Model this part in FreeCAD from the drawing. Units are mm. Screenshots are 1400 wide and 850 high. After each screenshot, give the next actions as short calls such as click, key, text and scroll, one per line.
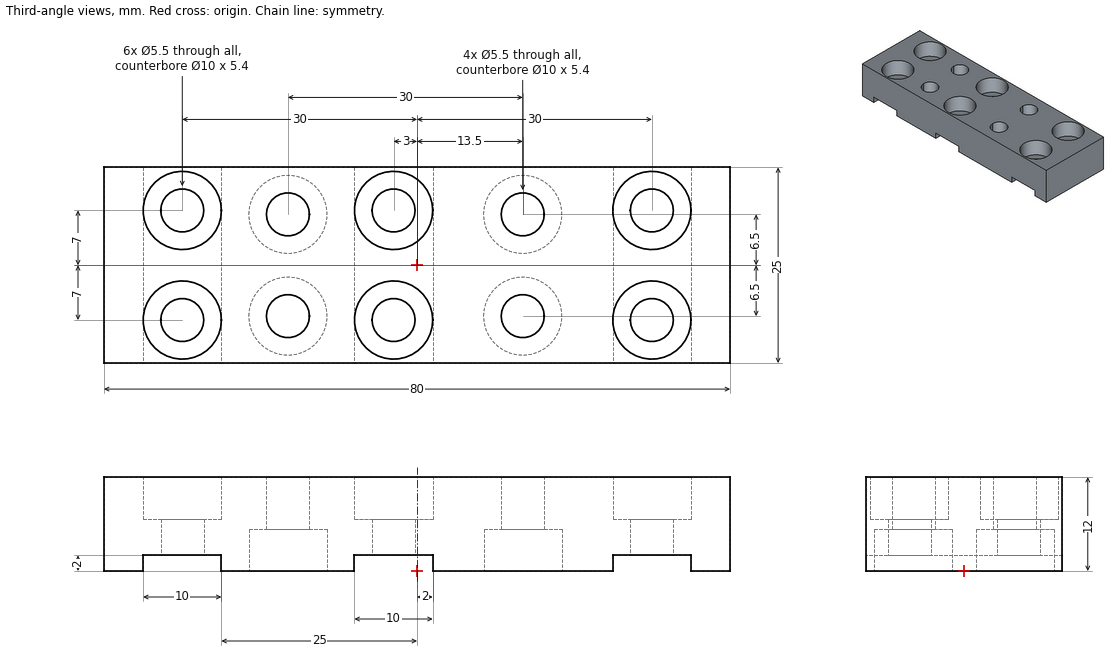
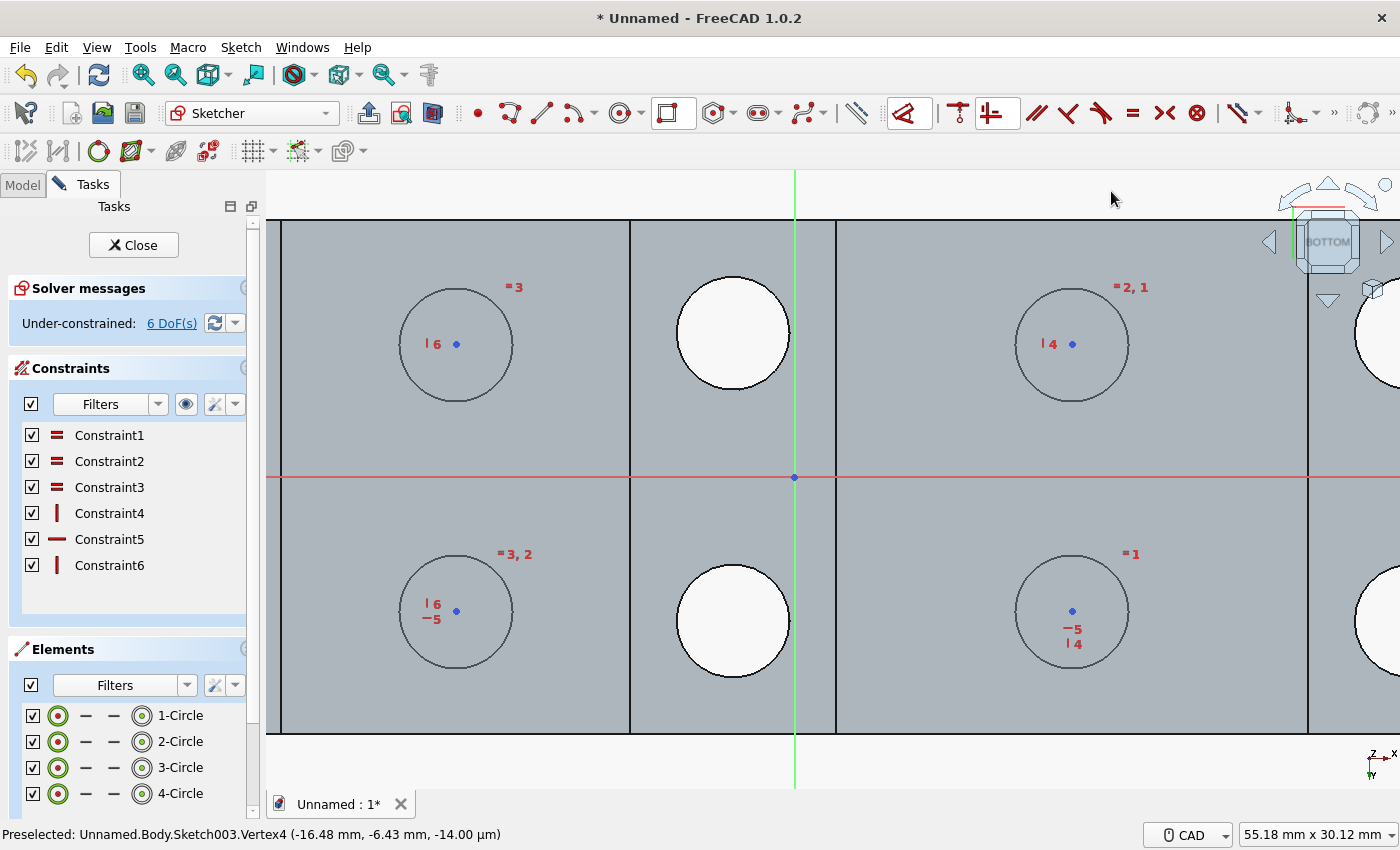
click(1072, 345)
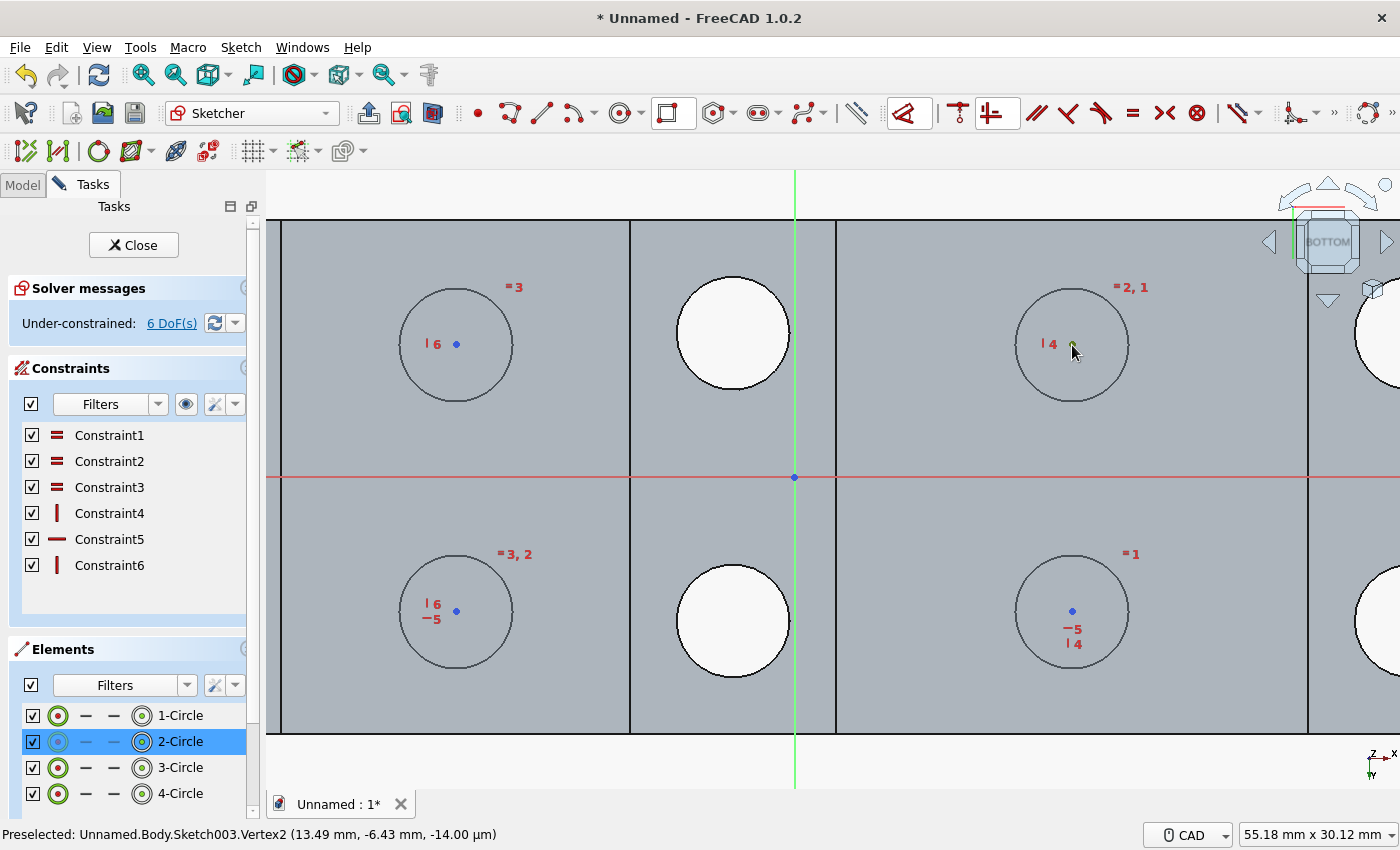
click(456, 345)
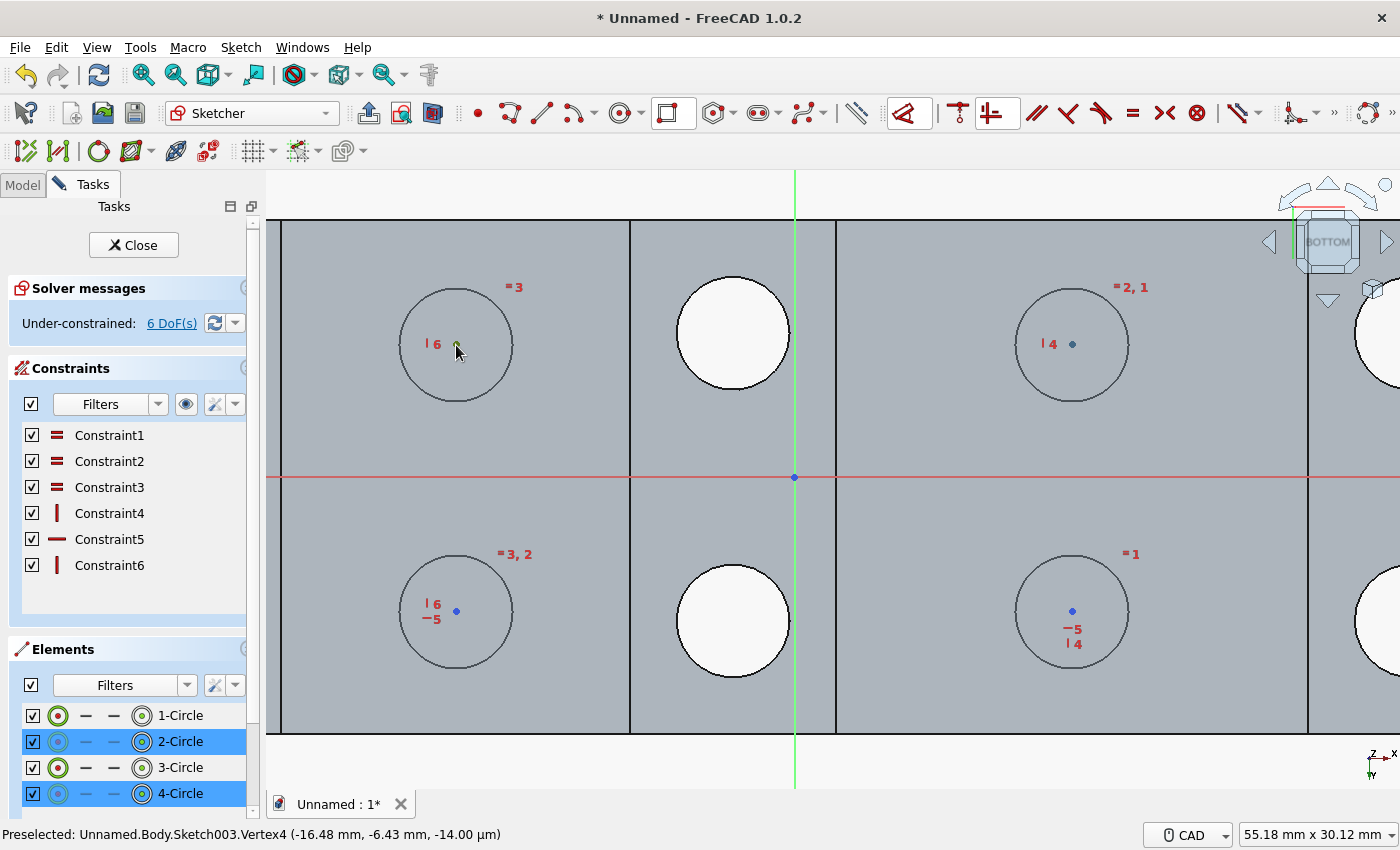
click(1014, 114)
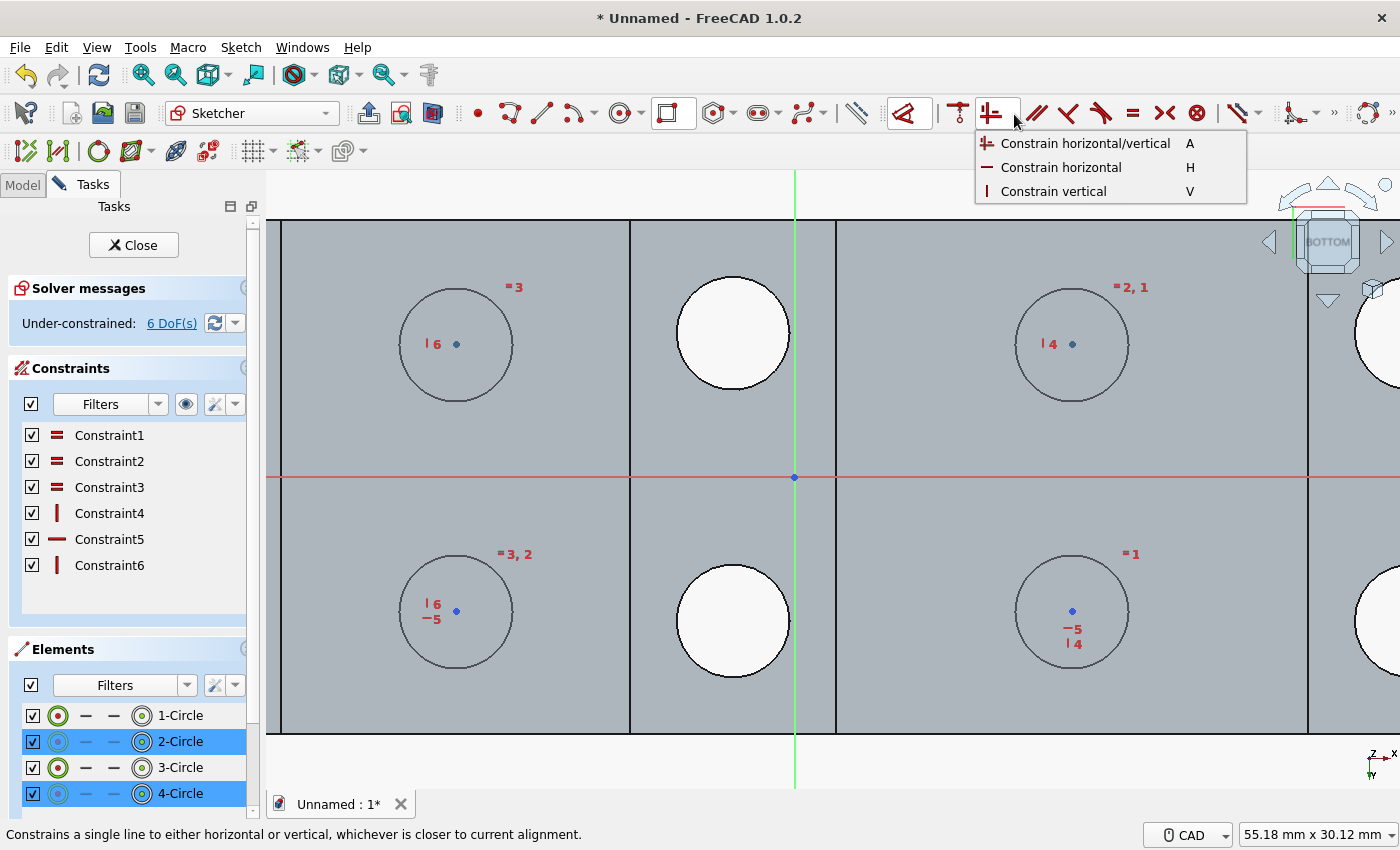
click(1111, 167)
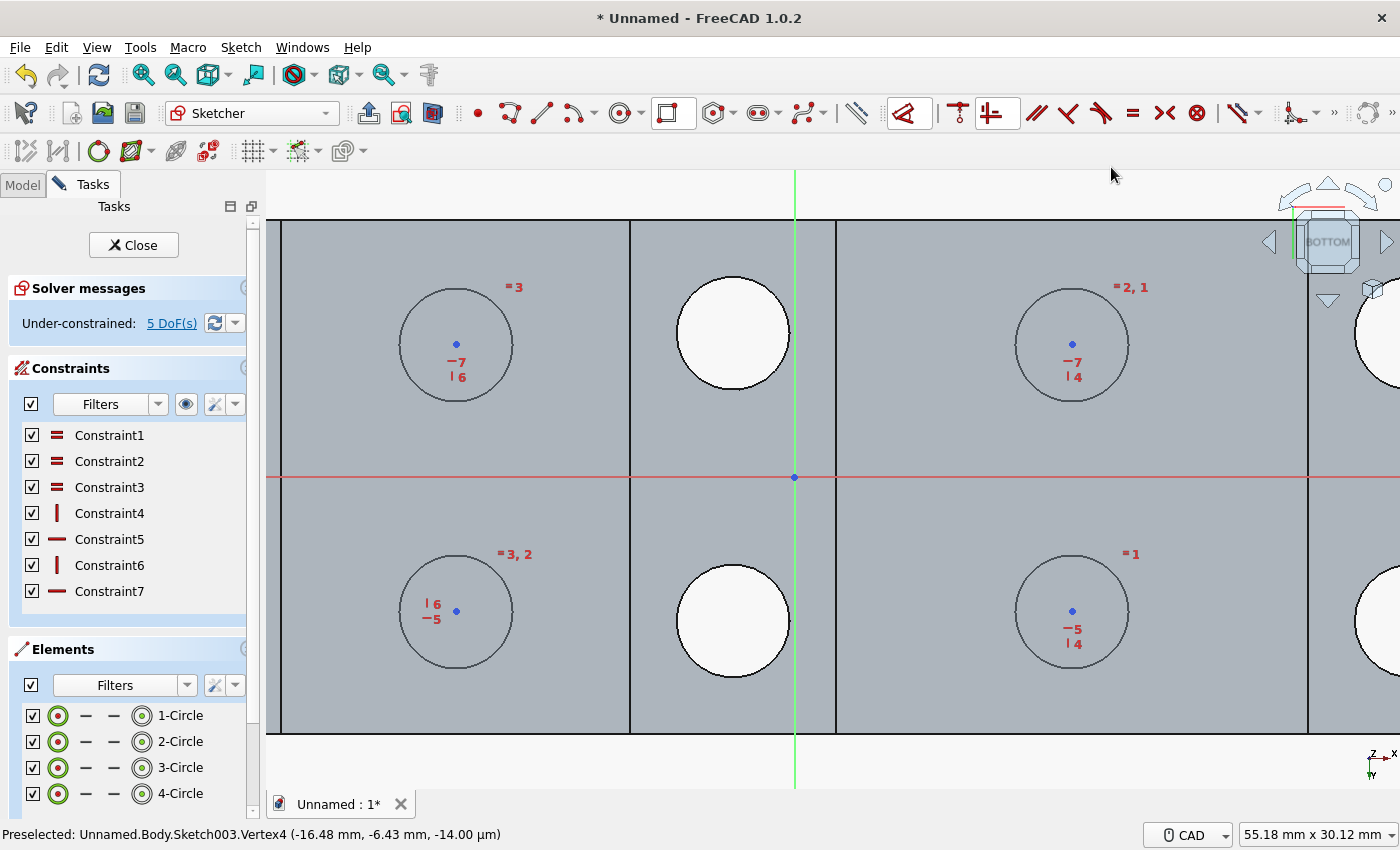
click(1112, 572)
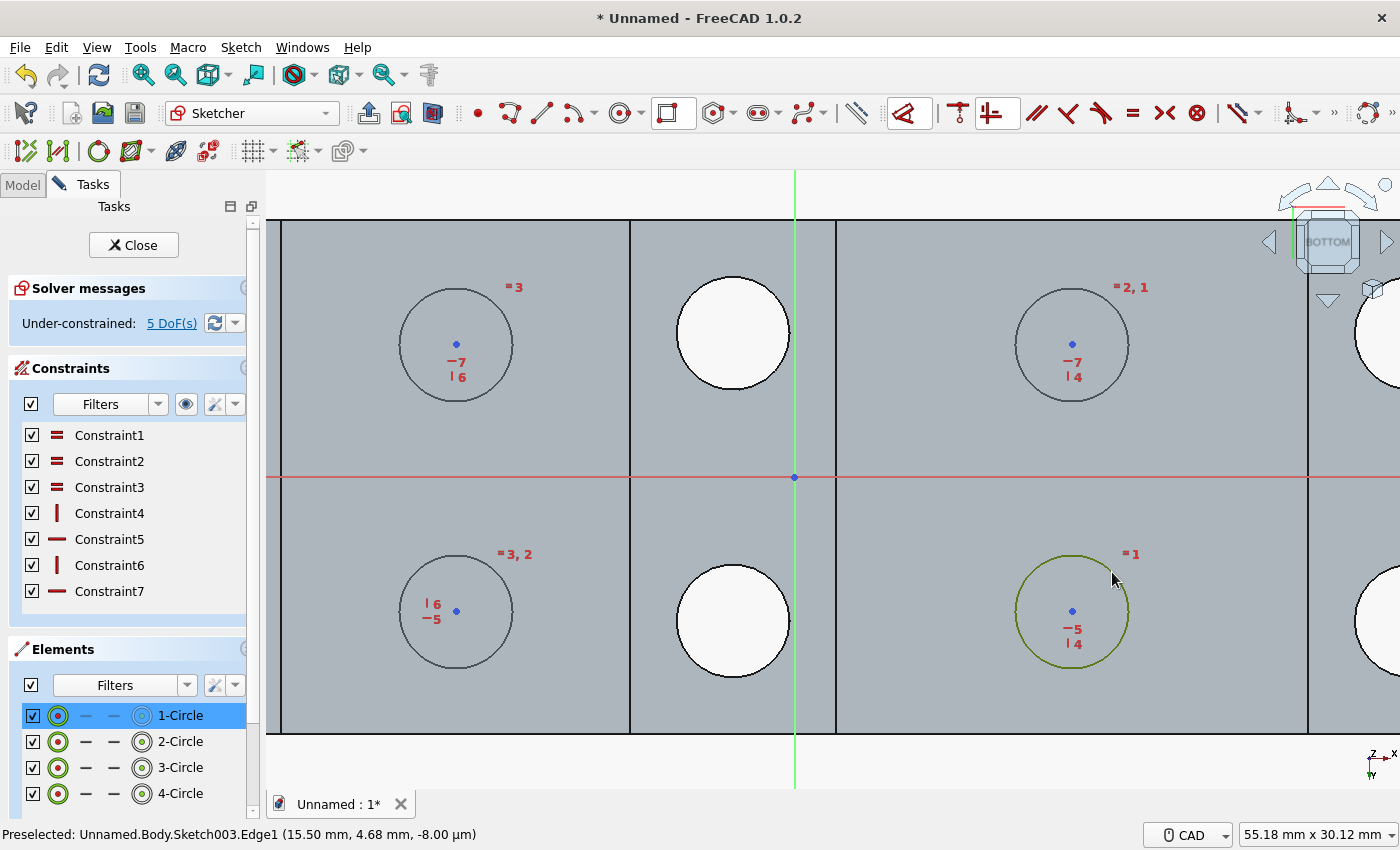
click(926, 114)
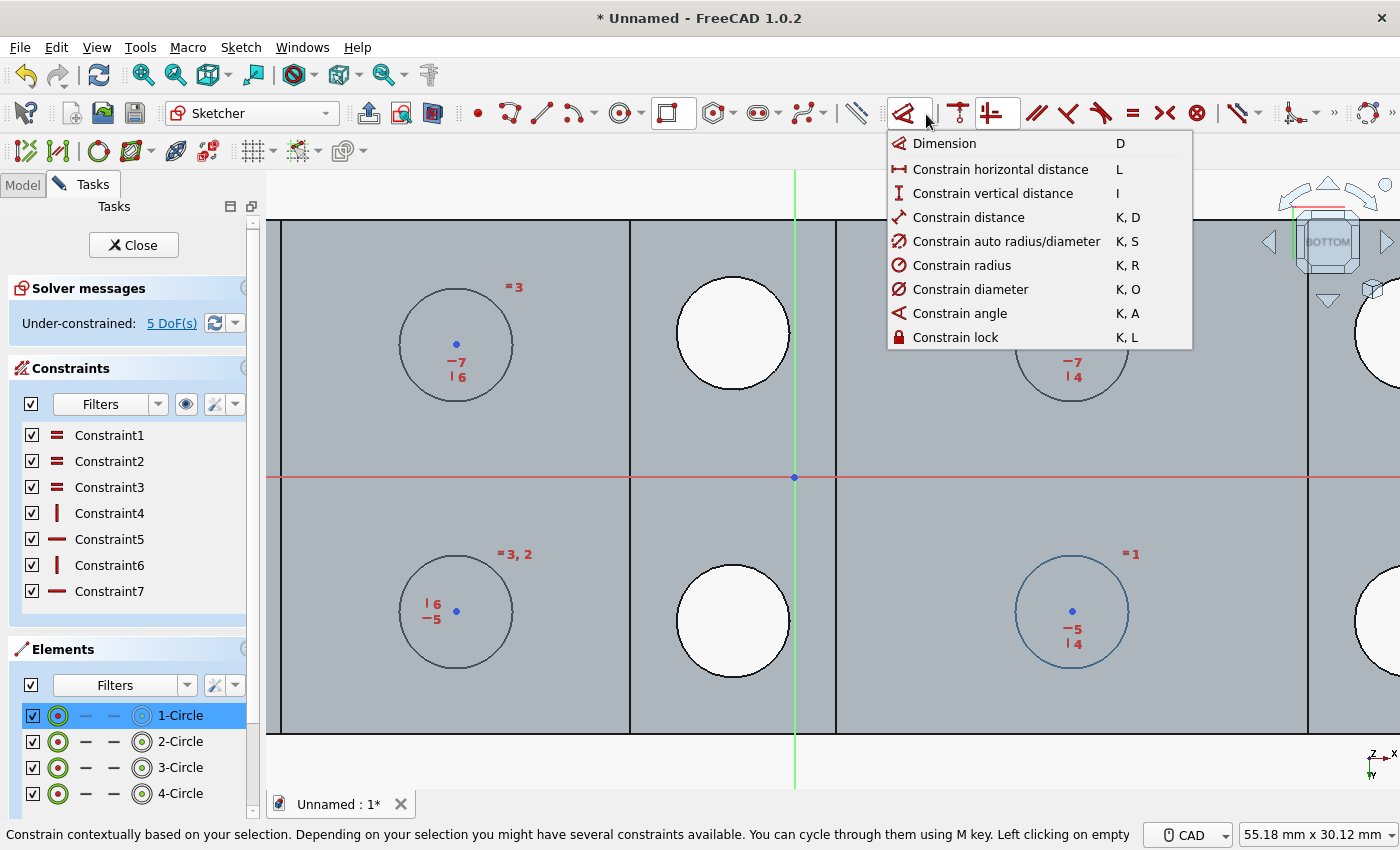
click(1040, 289)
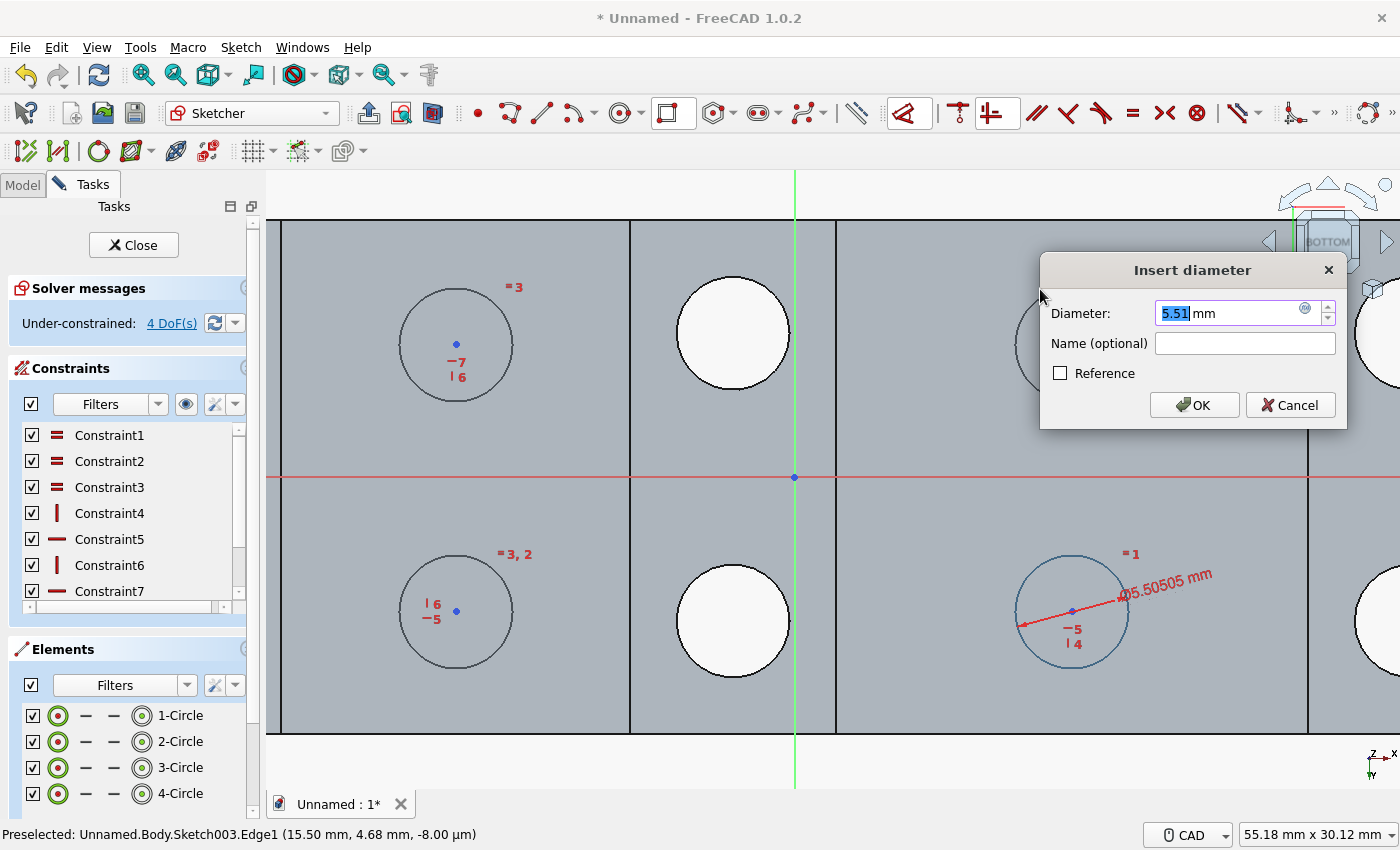
text(5.5)
key(Return)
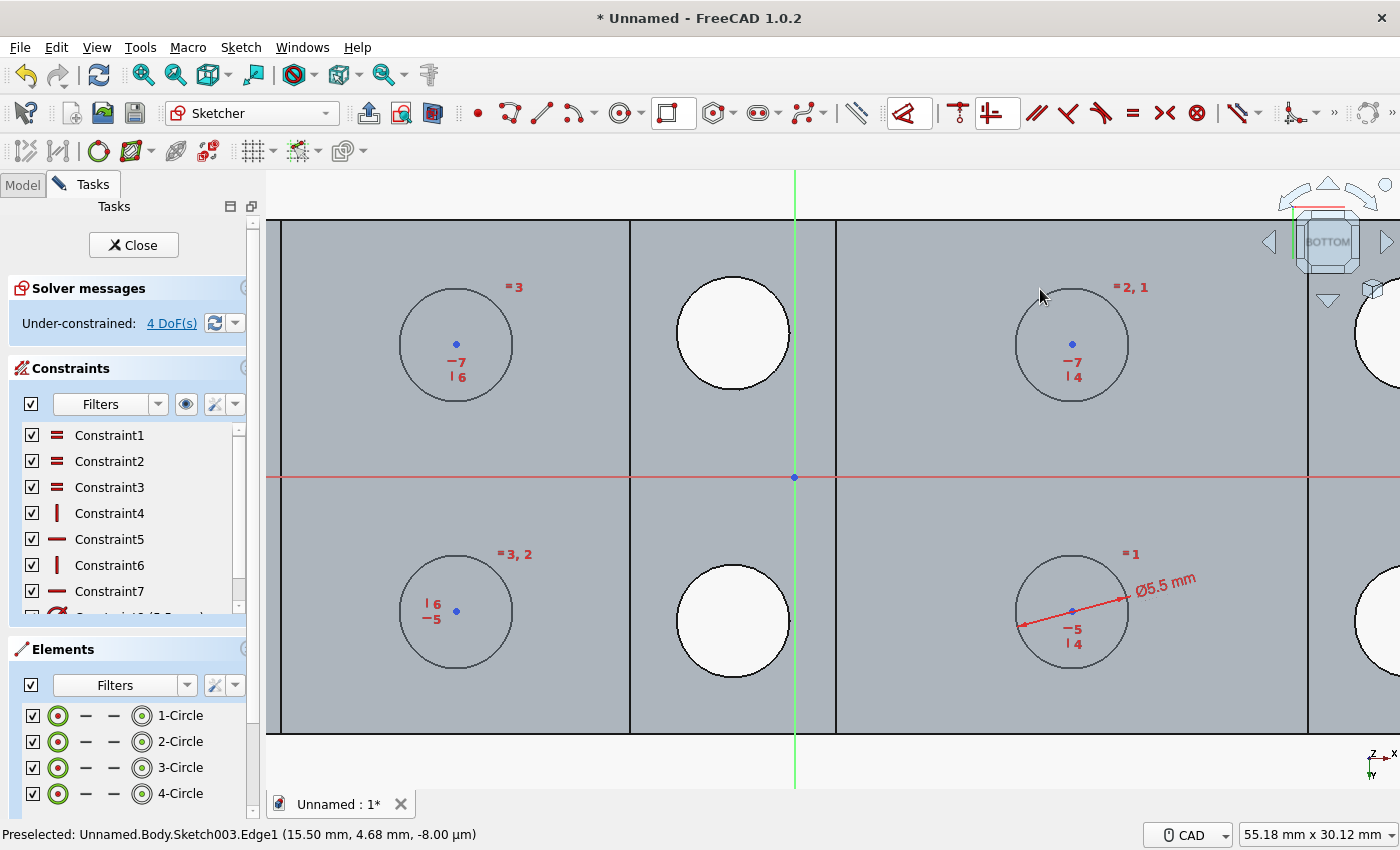
click(1072, 612)